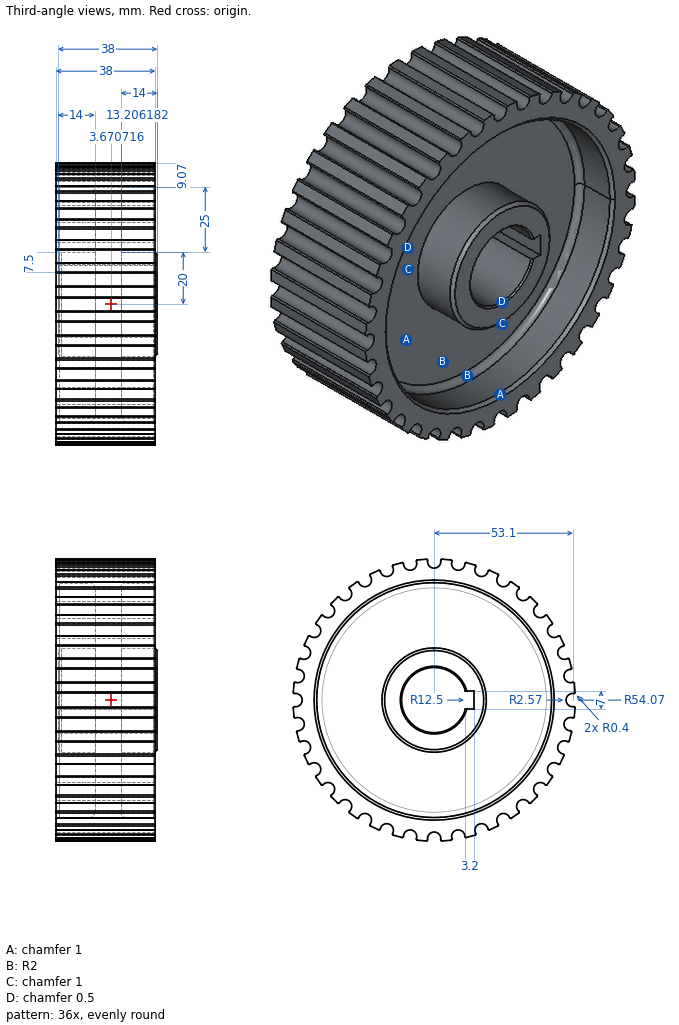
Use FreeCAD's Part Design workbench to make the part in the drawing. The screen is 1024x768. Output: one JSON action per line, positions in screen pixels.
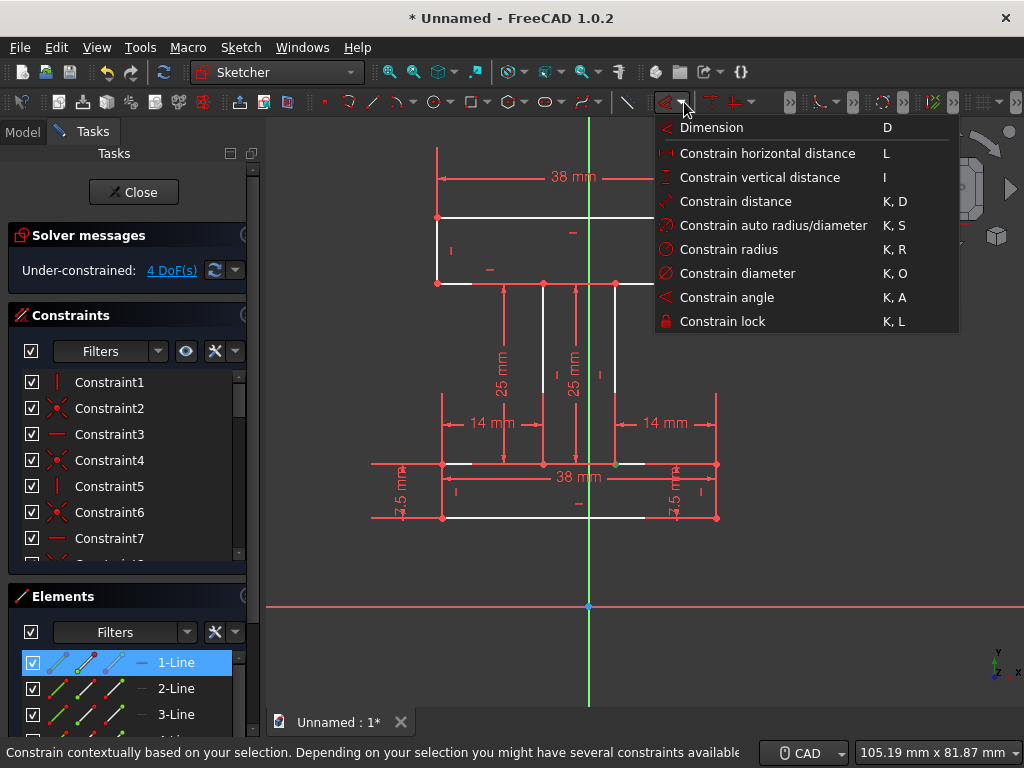
{"action": "left_click", "coordinate": [807, 177]}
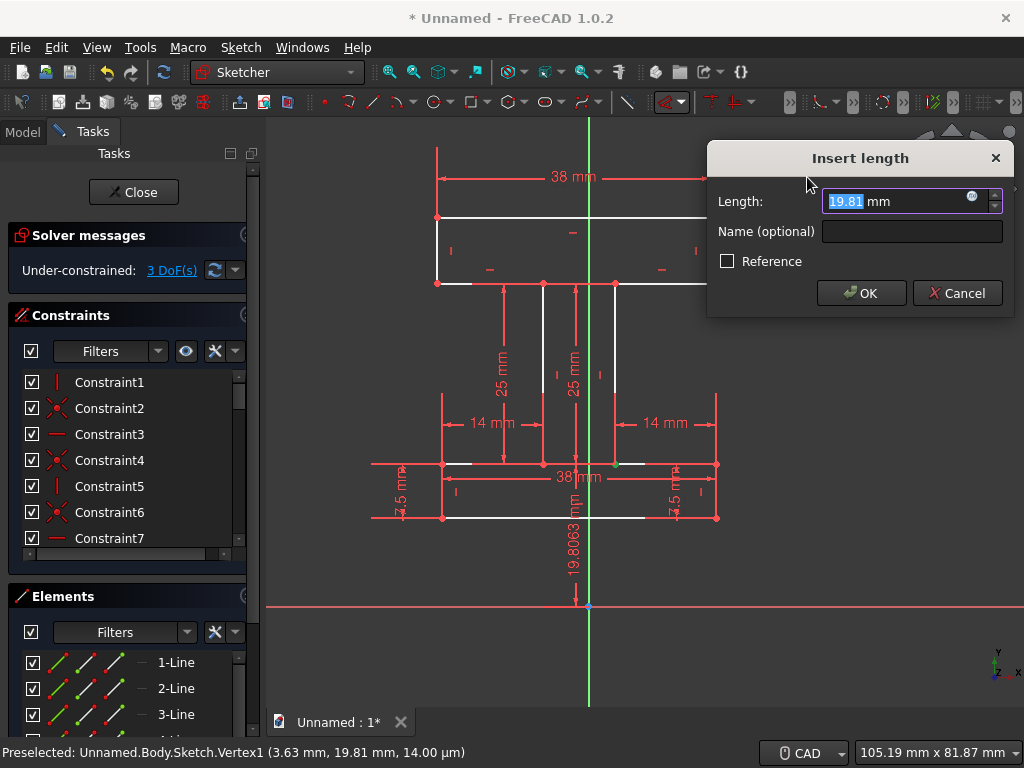
{"action": "type", "text": "20"}
{"action": "key", "text": "Return"}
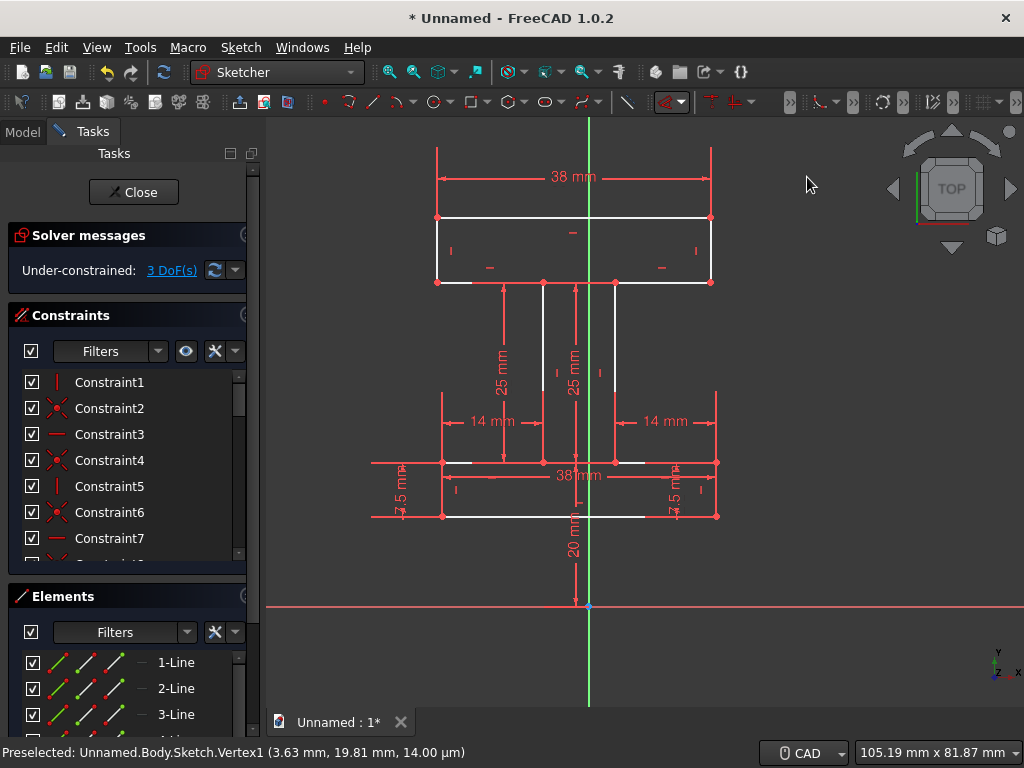
{"action": "left_click", "coordinate": [711, 263]}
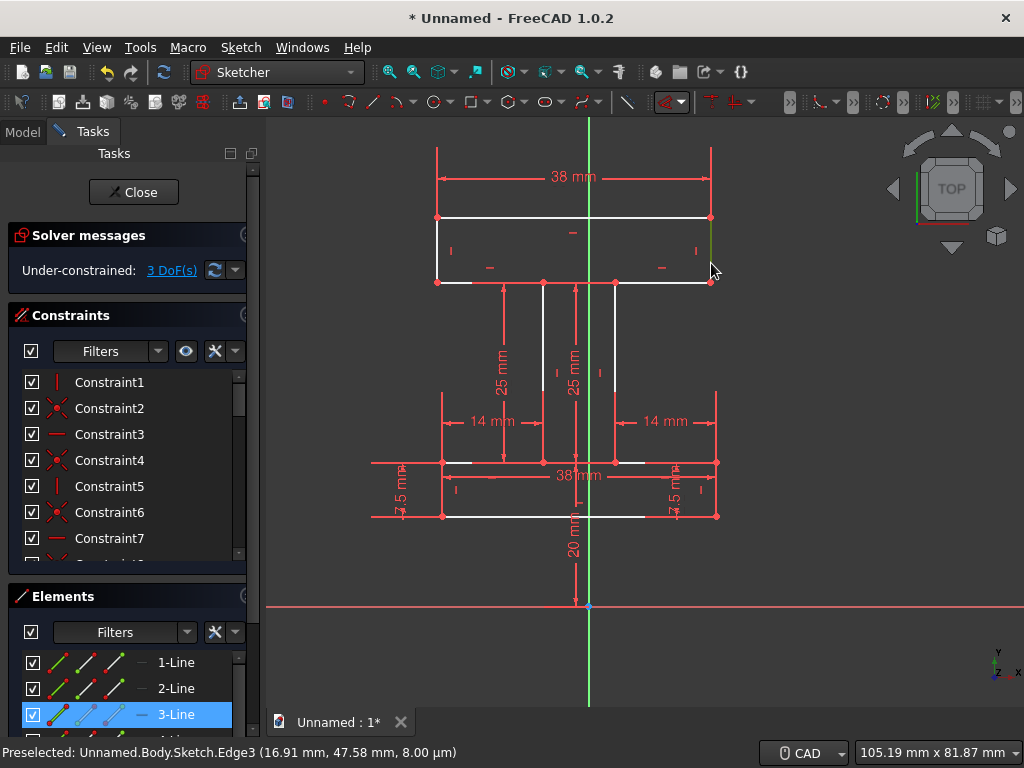
{"action": "key", "text": "i"}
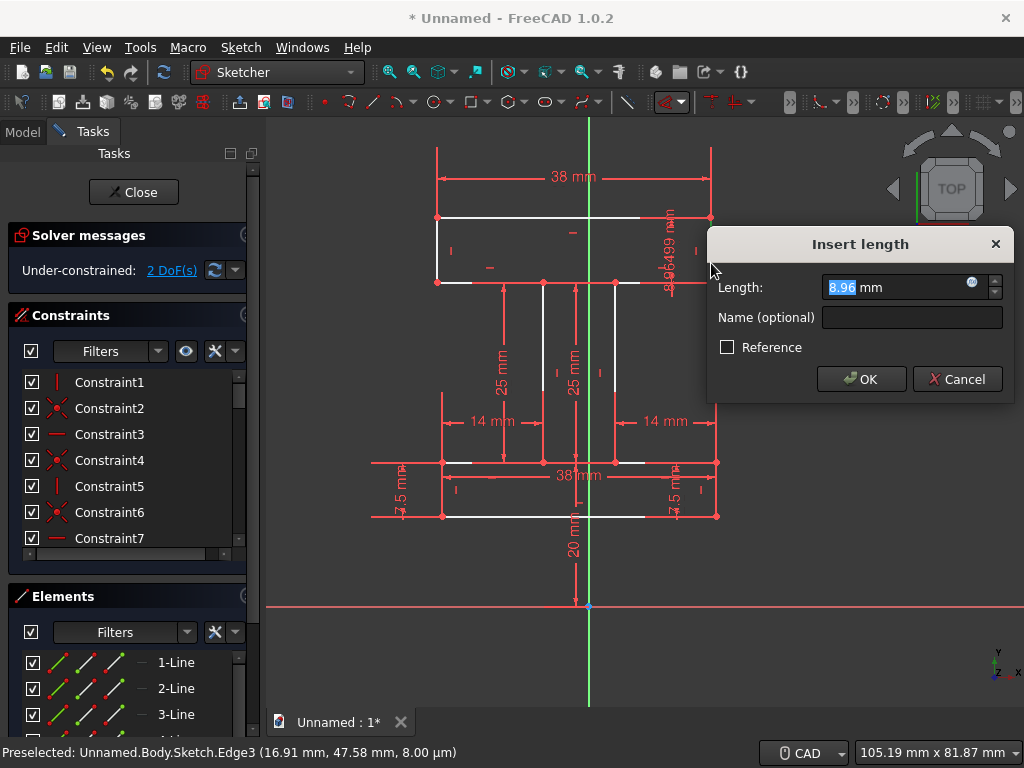
{"action": "type", "text": "9.07"}
{"action": "key", "text": "Return"}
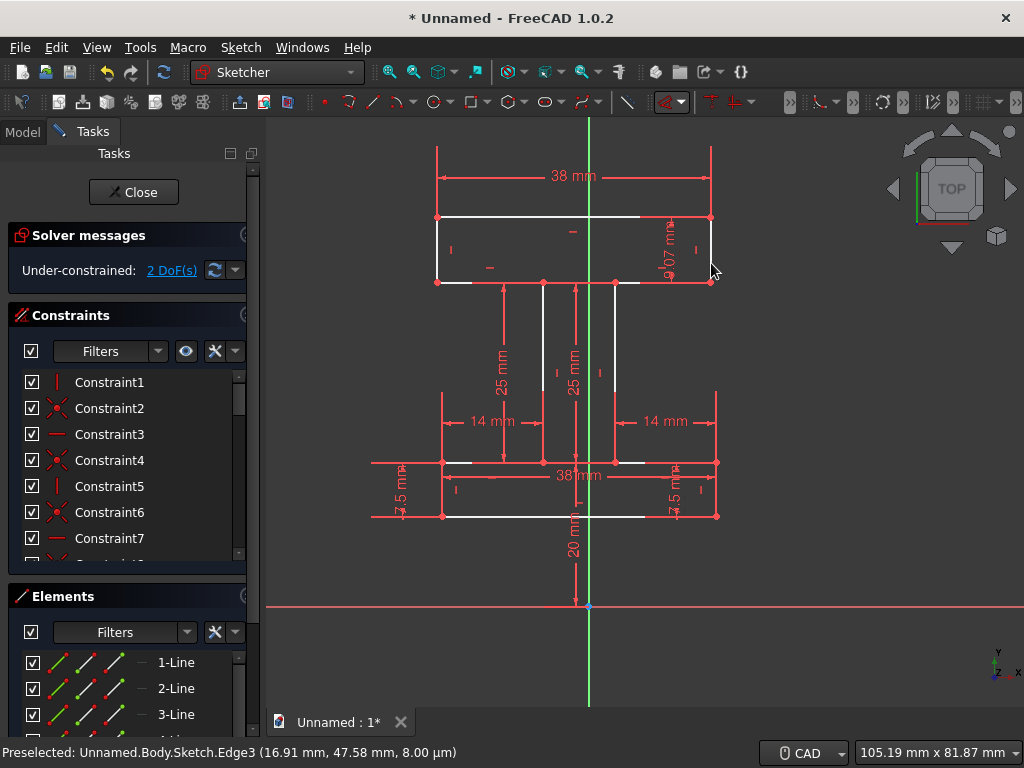
{"action": "left_click", "coordinate": [644, 283]}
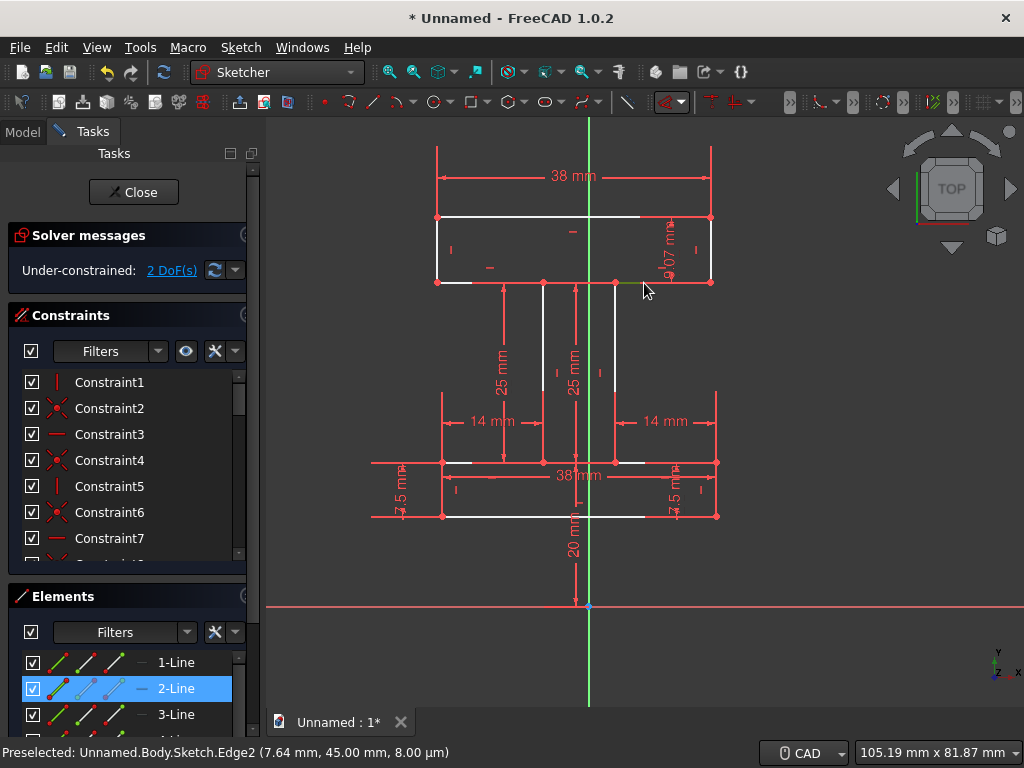
{"action": "left_click", "coordinate": [684, 102]}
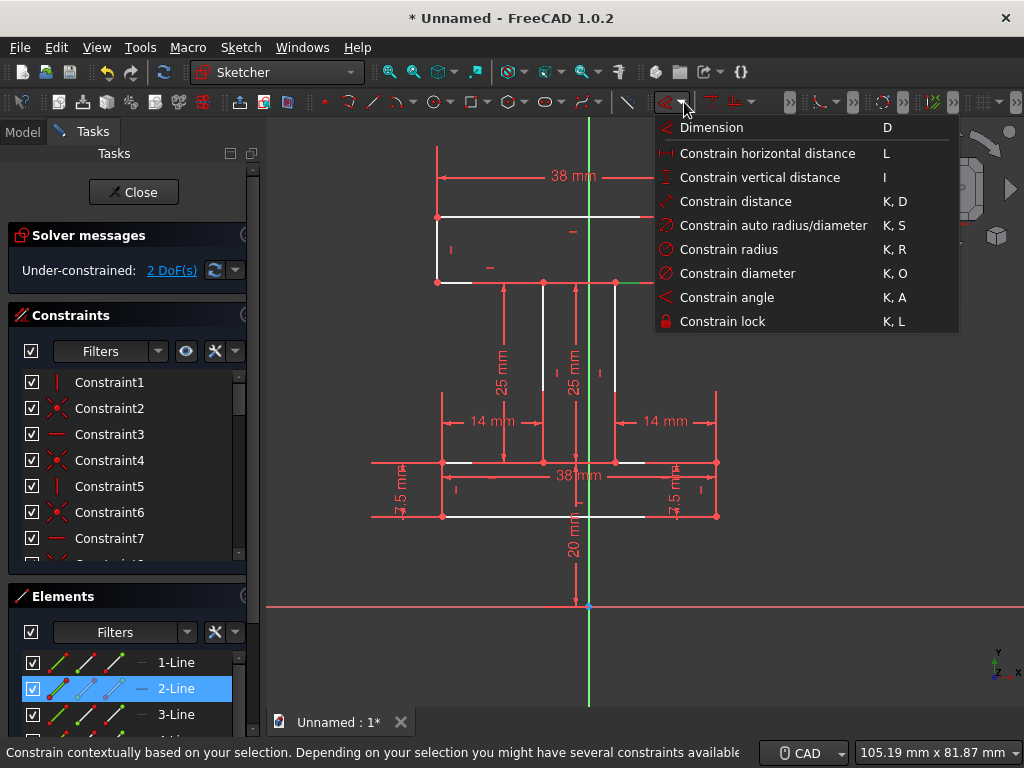
{"action": "left_click", "coordinate": [807, 153]}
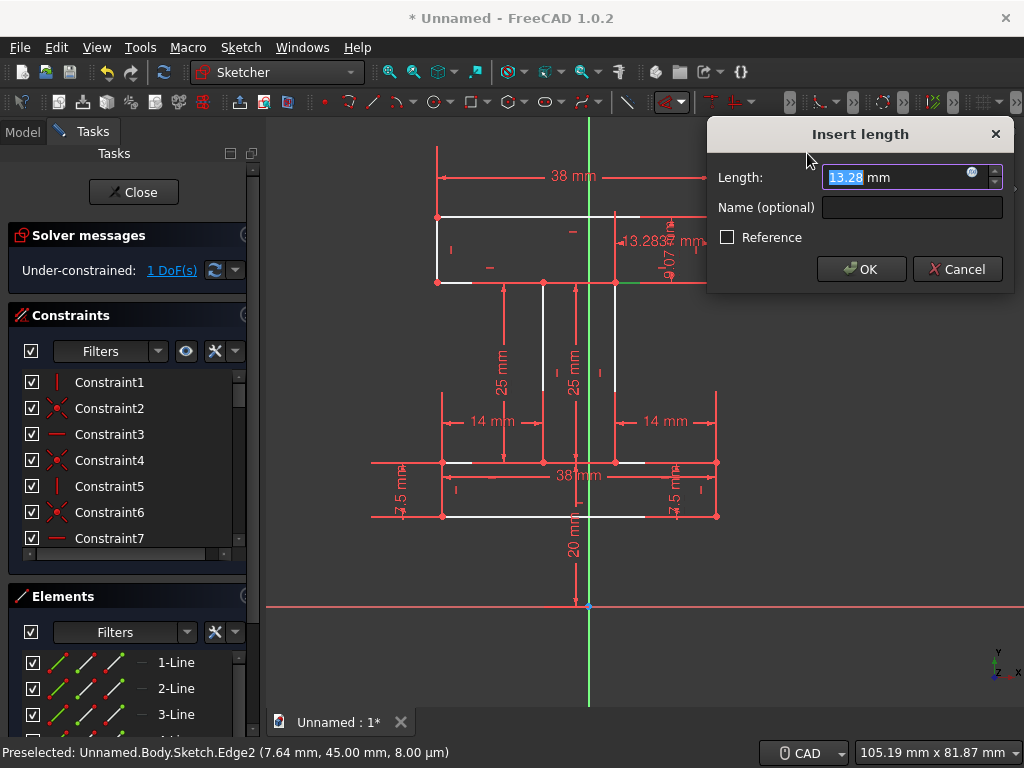
{"action": "type", "text": "13.206182"}
{"action": "key", "text": "Return"}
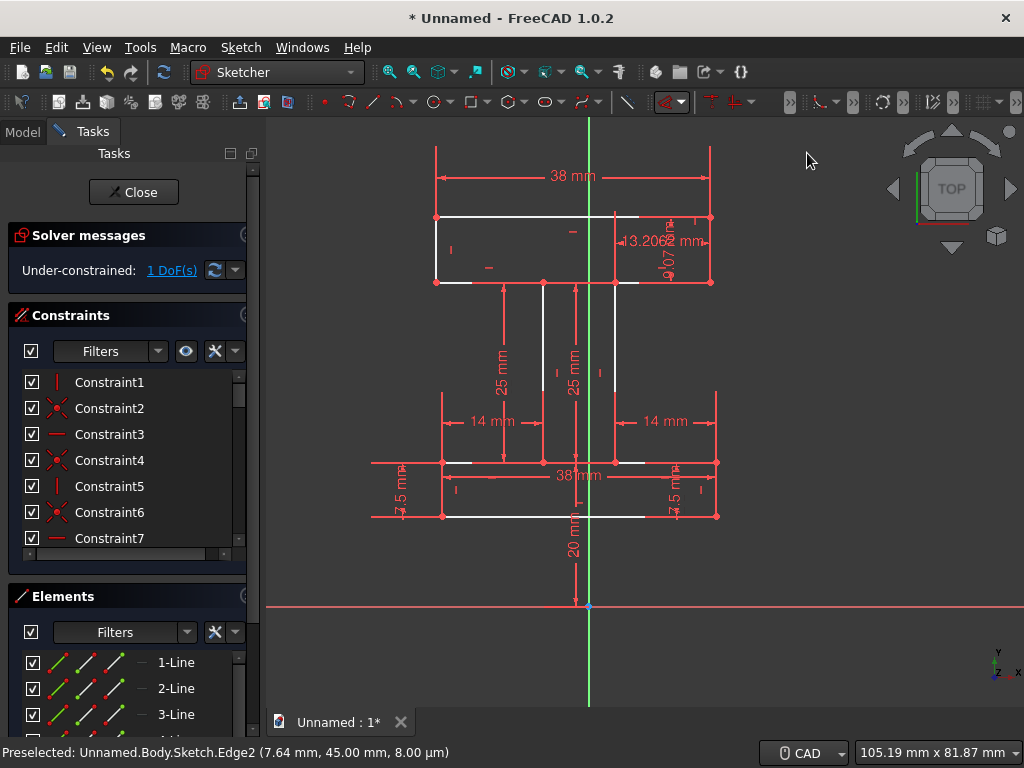
{"action": "scroll", "coordinate": [615, 463], "scroll_direction": "up", "scroll_amount": 3}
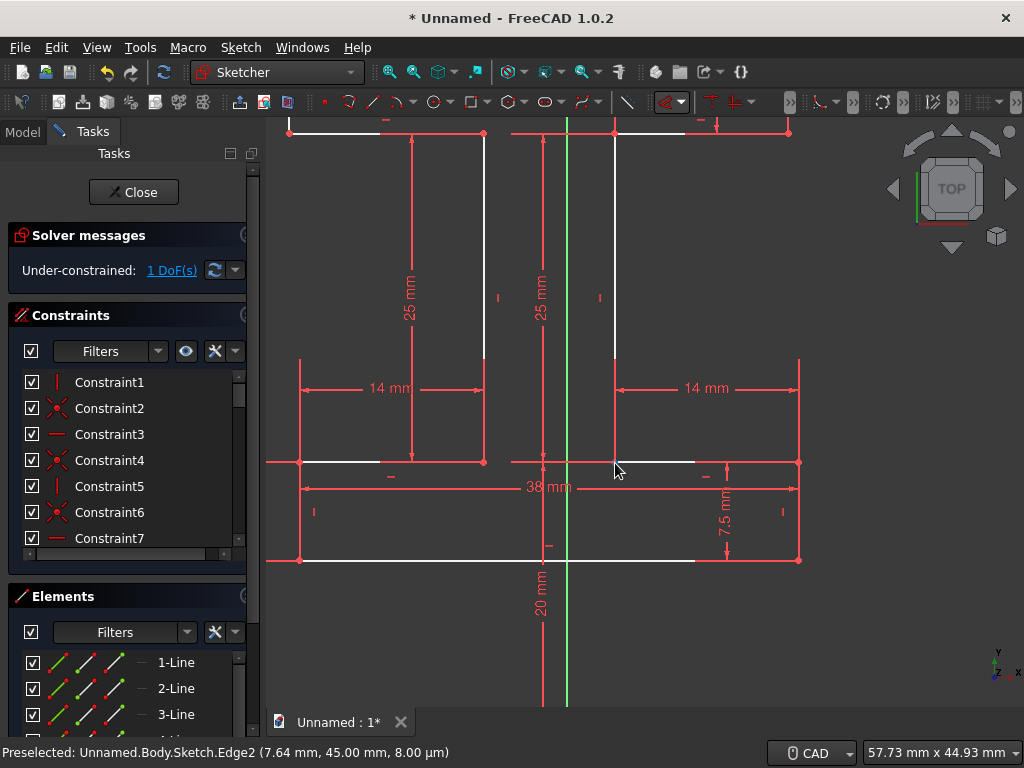
{"action": "left_click", "coordinate": [615, 462]}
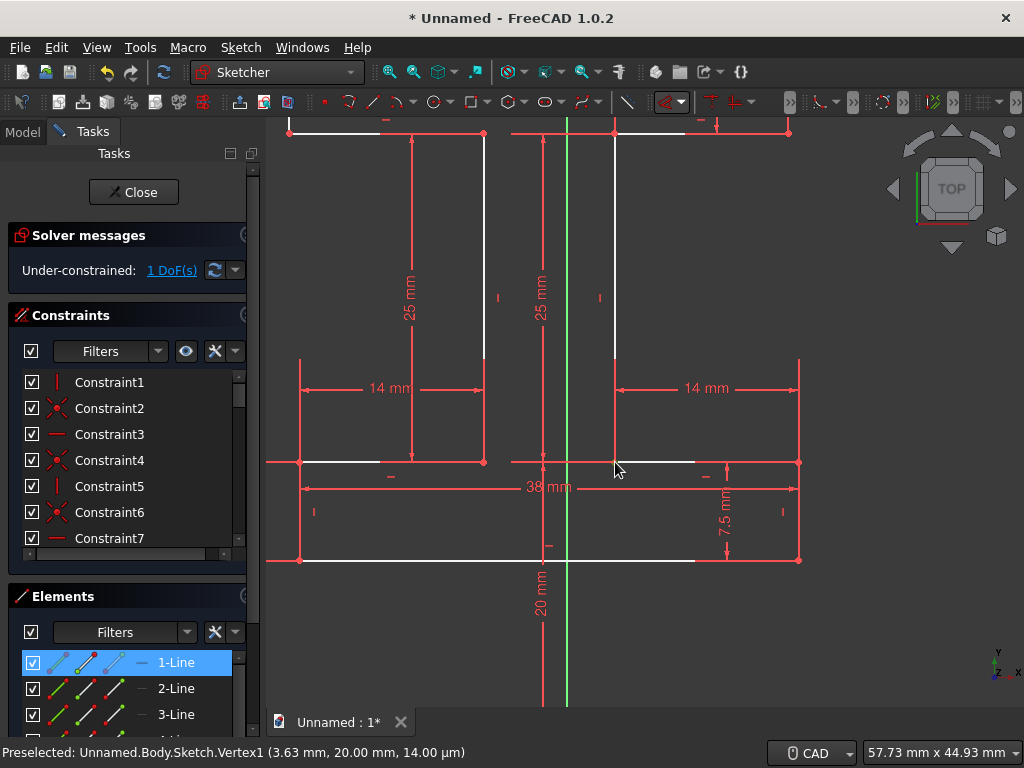
{"action": "left_click", "coordinate": [684, 102]}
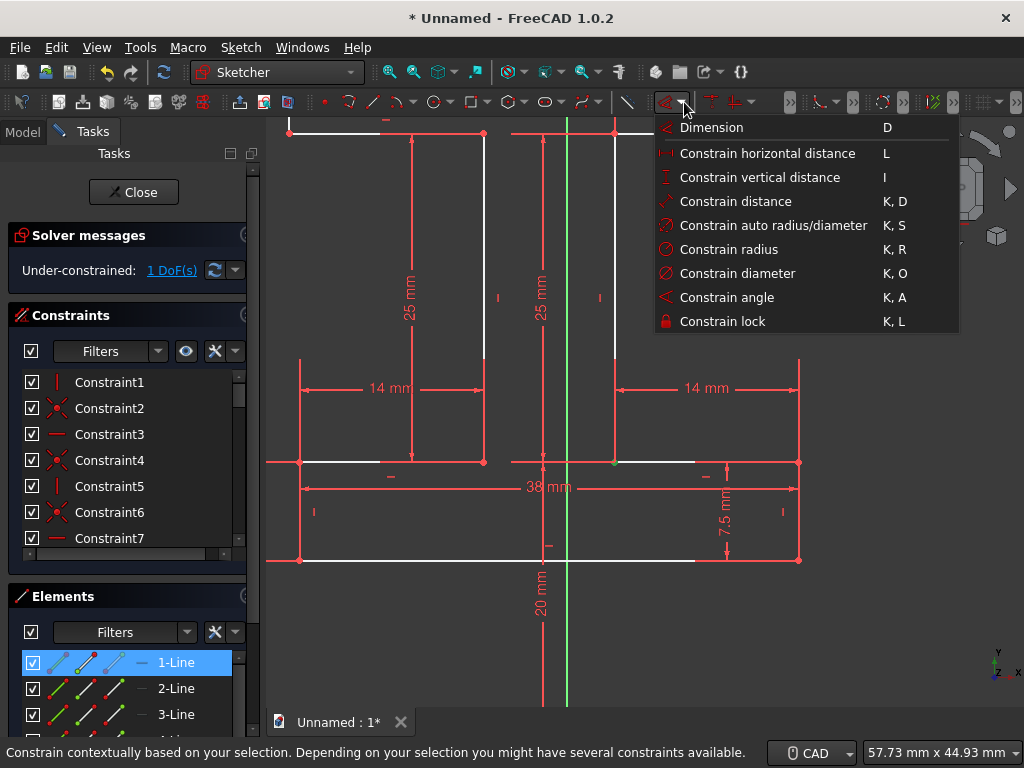
{"action": "left_click", "coordinate": [807, 153]}